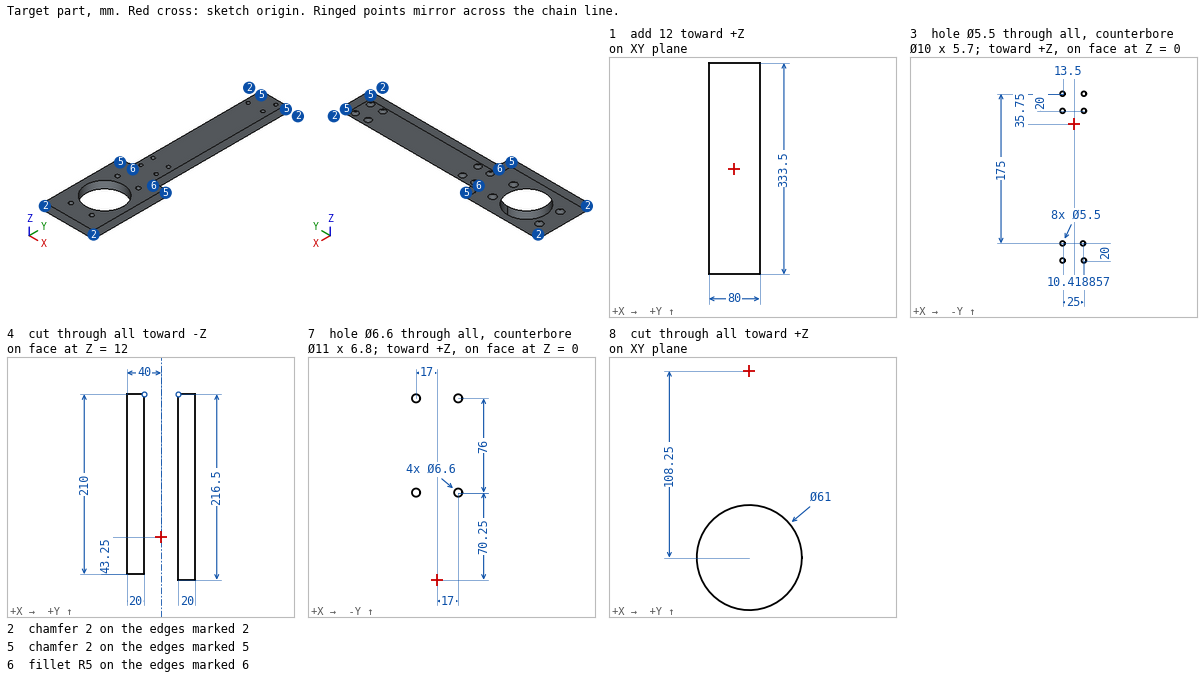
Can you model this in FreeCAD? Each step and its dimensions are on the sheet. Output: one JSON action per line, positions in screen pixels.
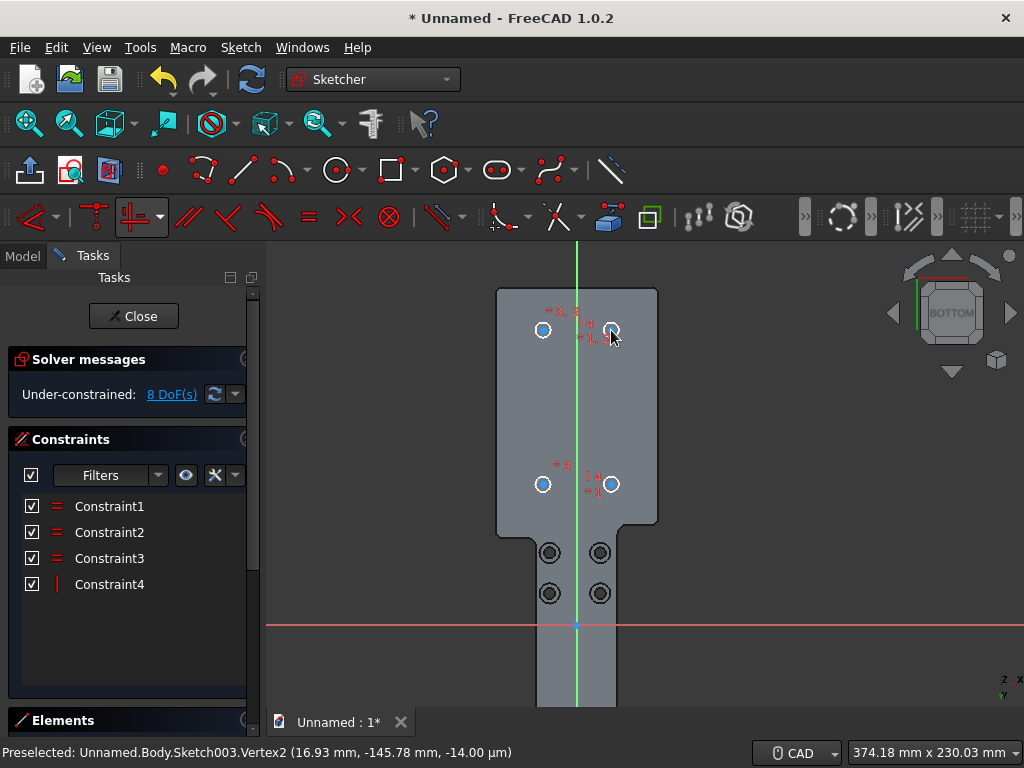
{"action": "left_click", "coordinate": [611, 330]}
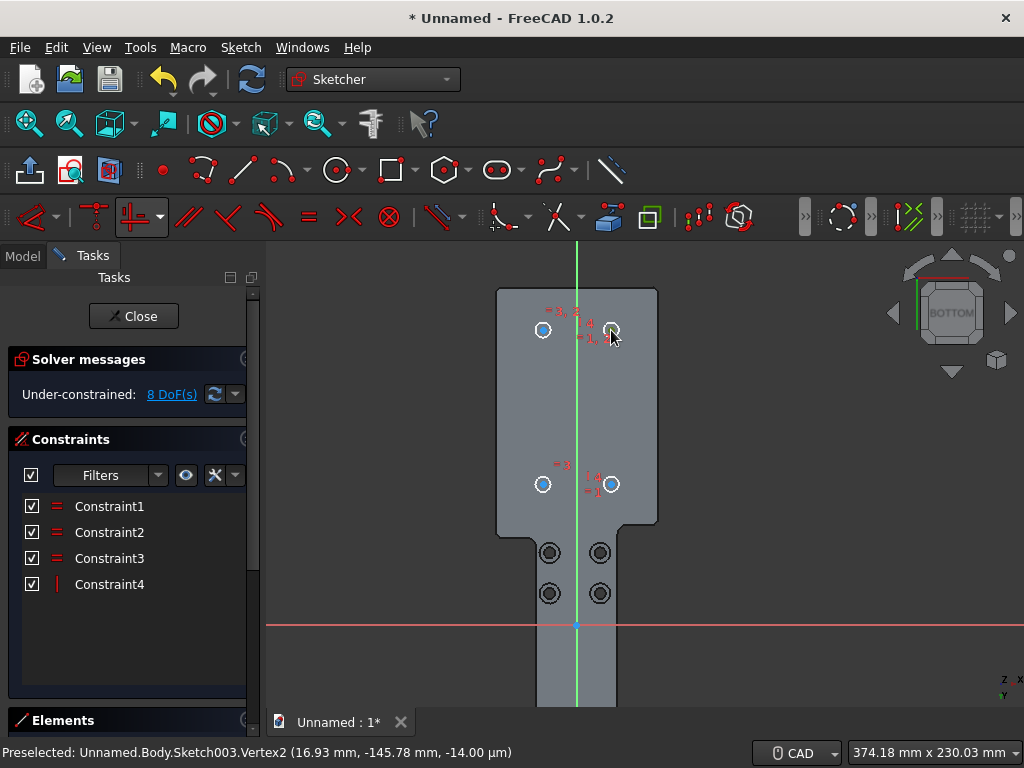
{"action": "left_click", "coordinate": [543, 330]}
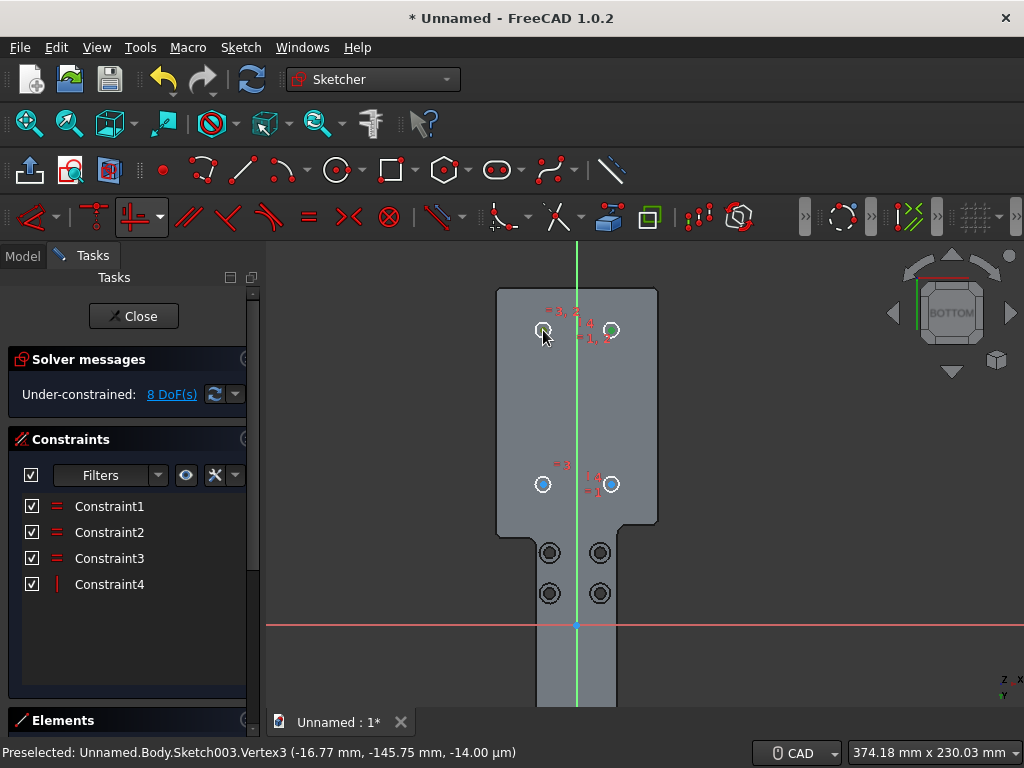
{"action": "key", "text": "h"}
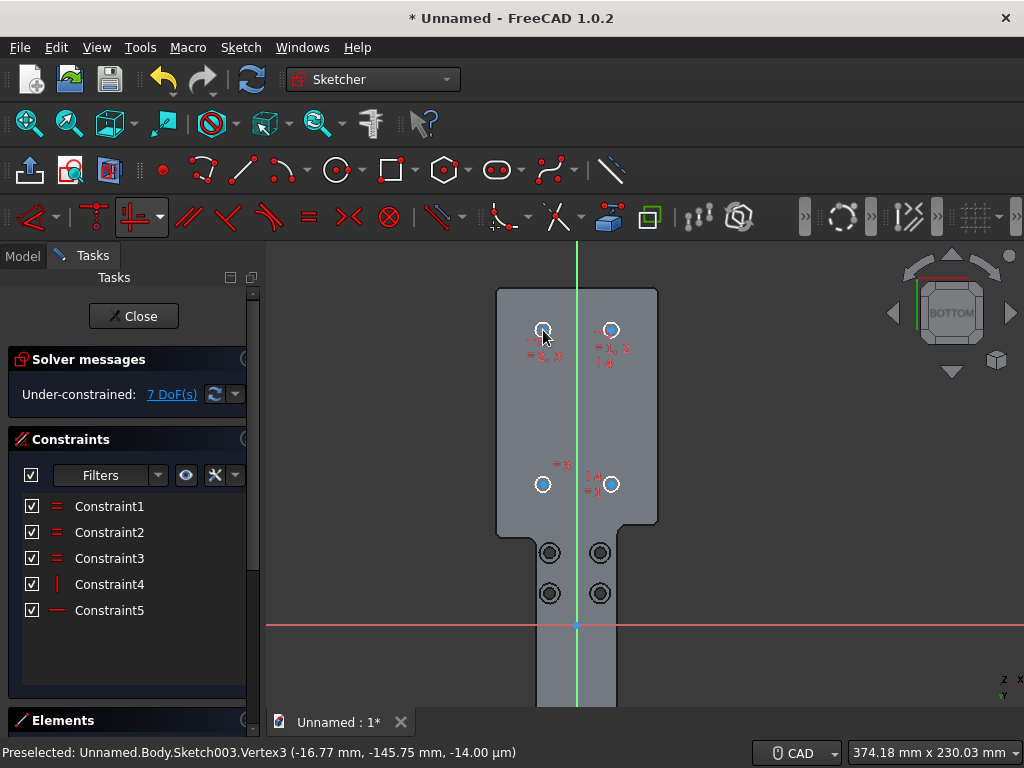
{"action": "left_click", "coordinate": [543, 330]}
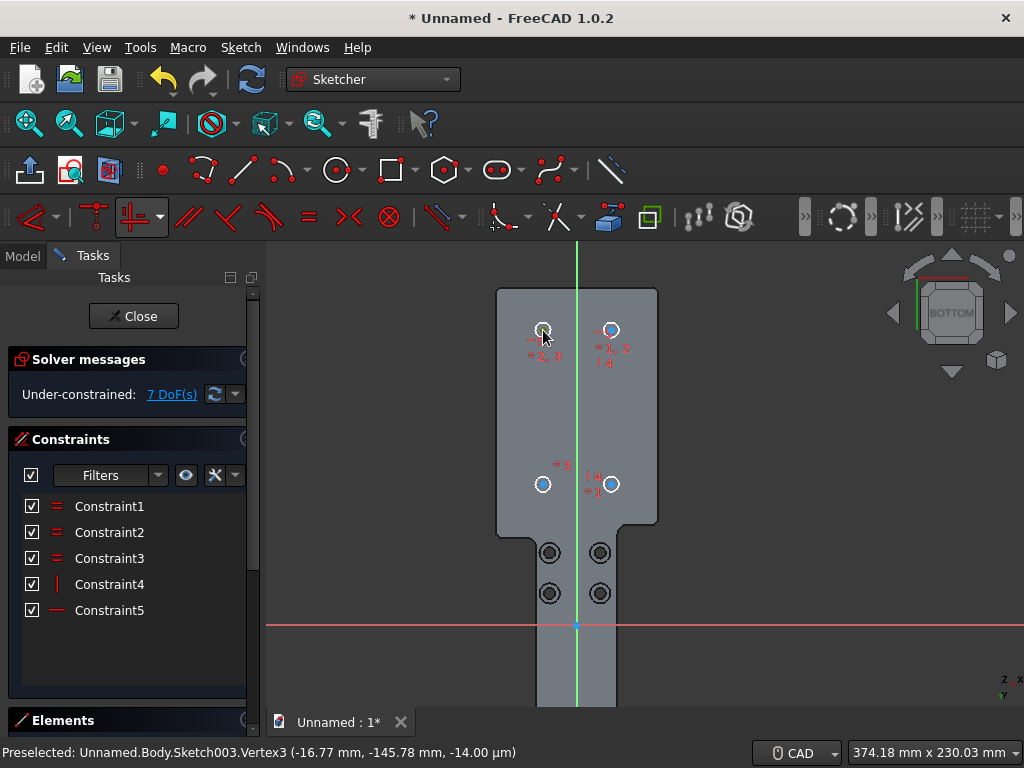
{"action": "left_click", "coordinate": [543, 484]}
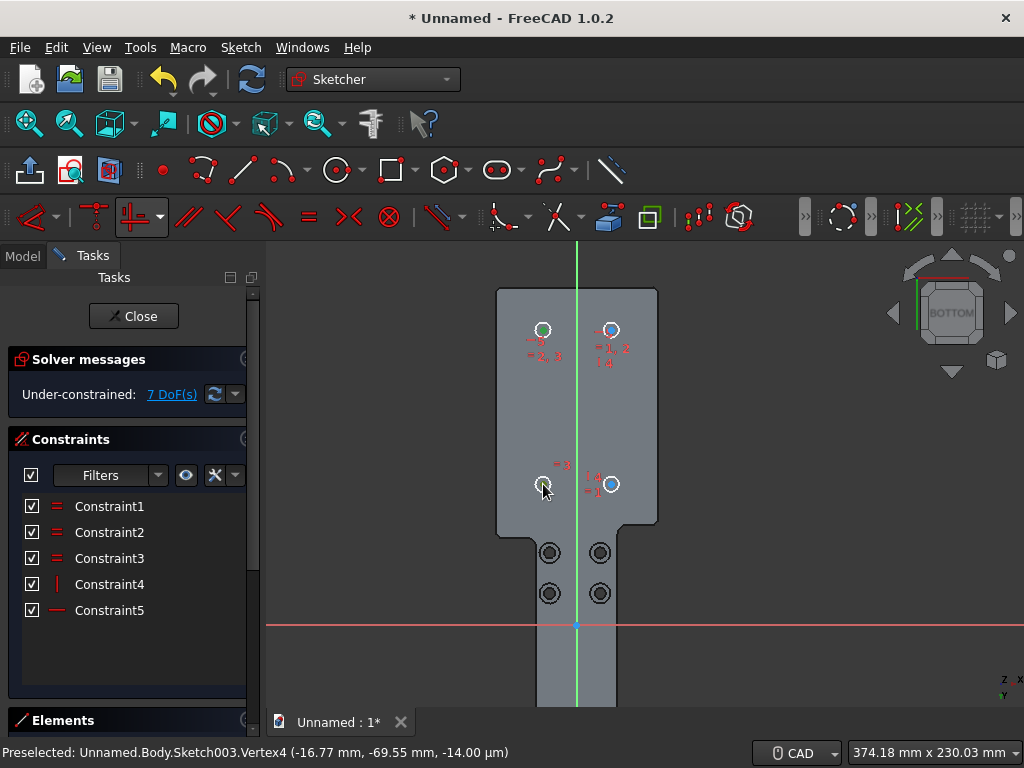
{"action": "key", "text": "v"}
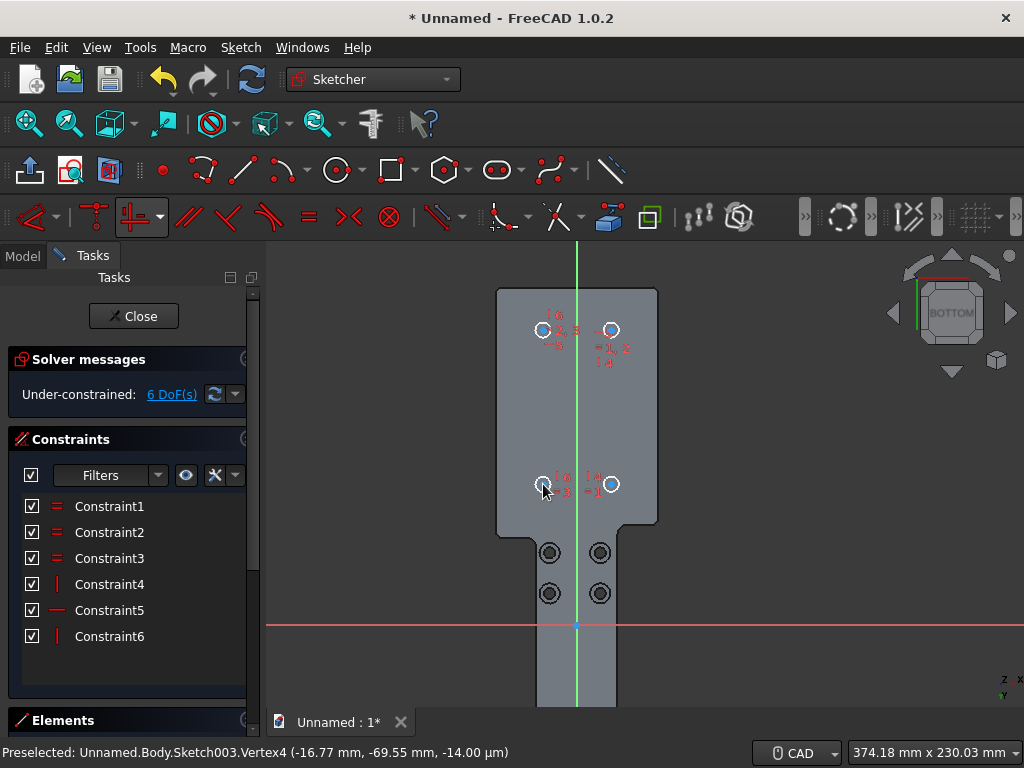
{"action": "left_click", "coordinate": [611, 484]}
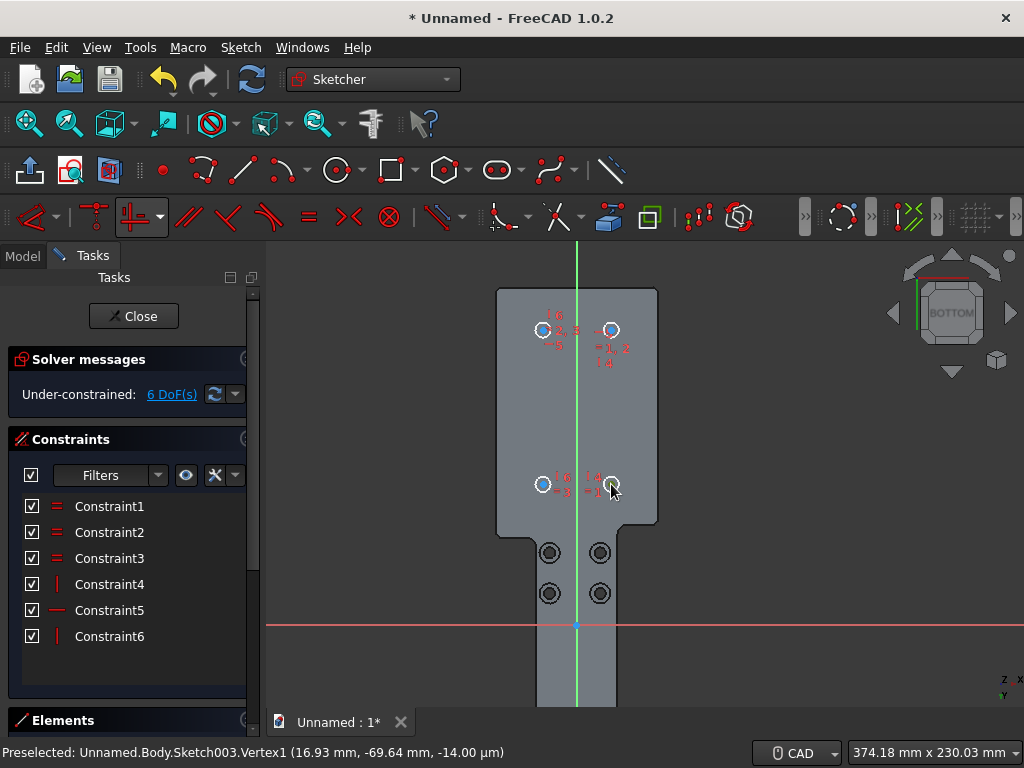
{"action": "left_click", "coordinate": [543, 484]}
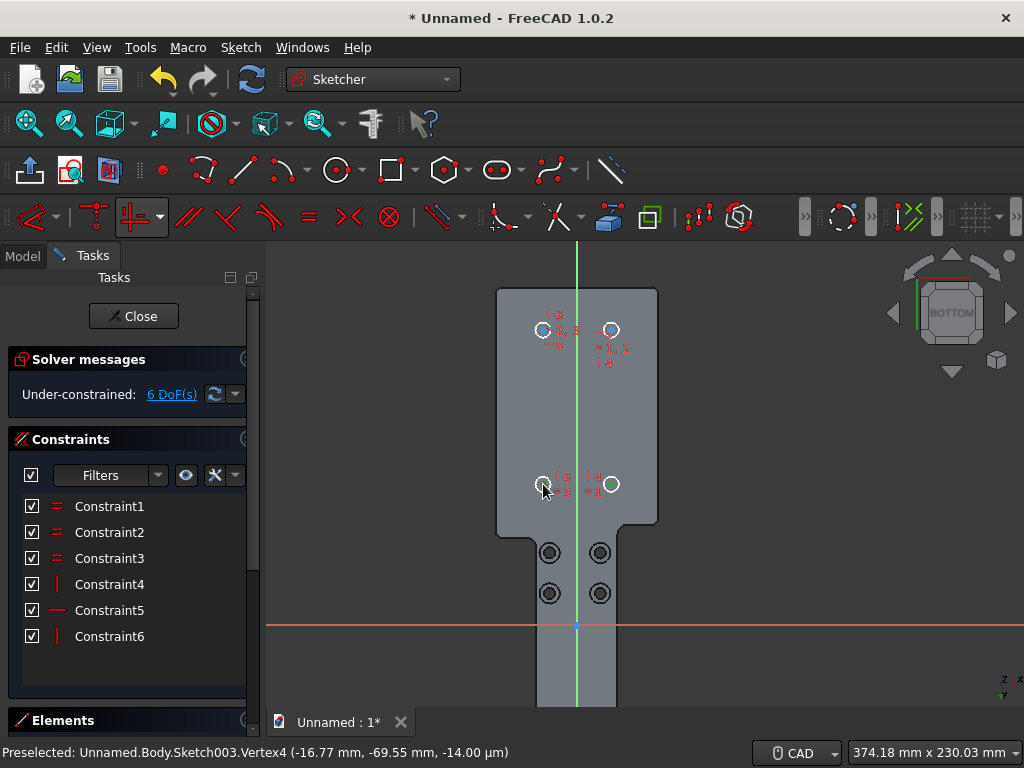
{"action": "key", "text": "h"}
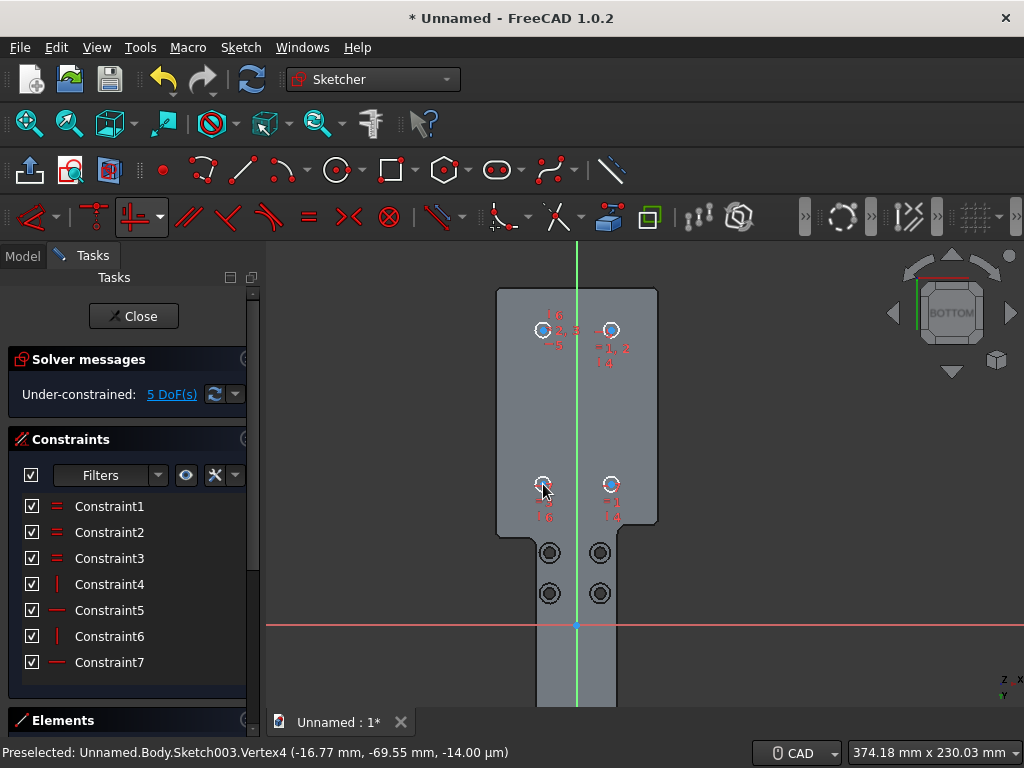
{"action": "left_click", "coordinate": [32, 218]}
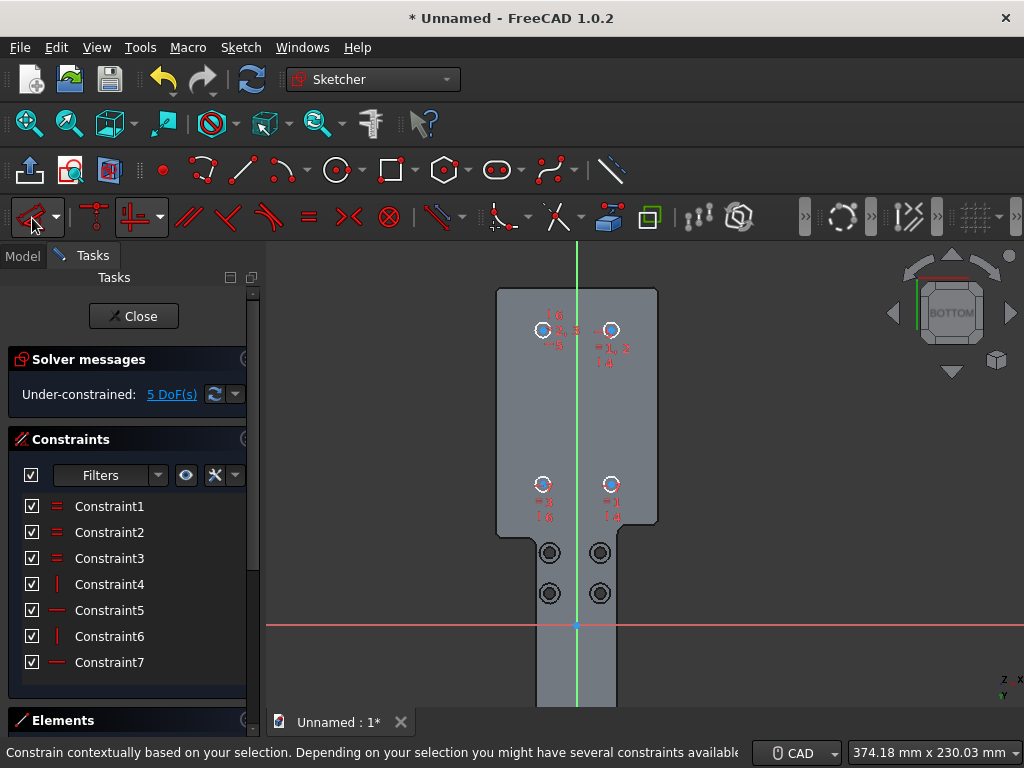
{"action": "scroll", "coordinate": [617, 490], "scroll_direction": "up", "scroll_amount": 6}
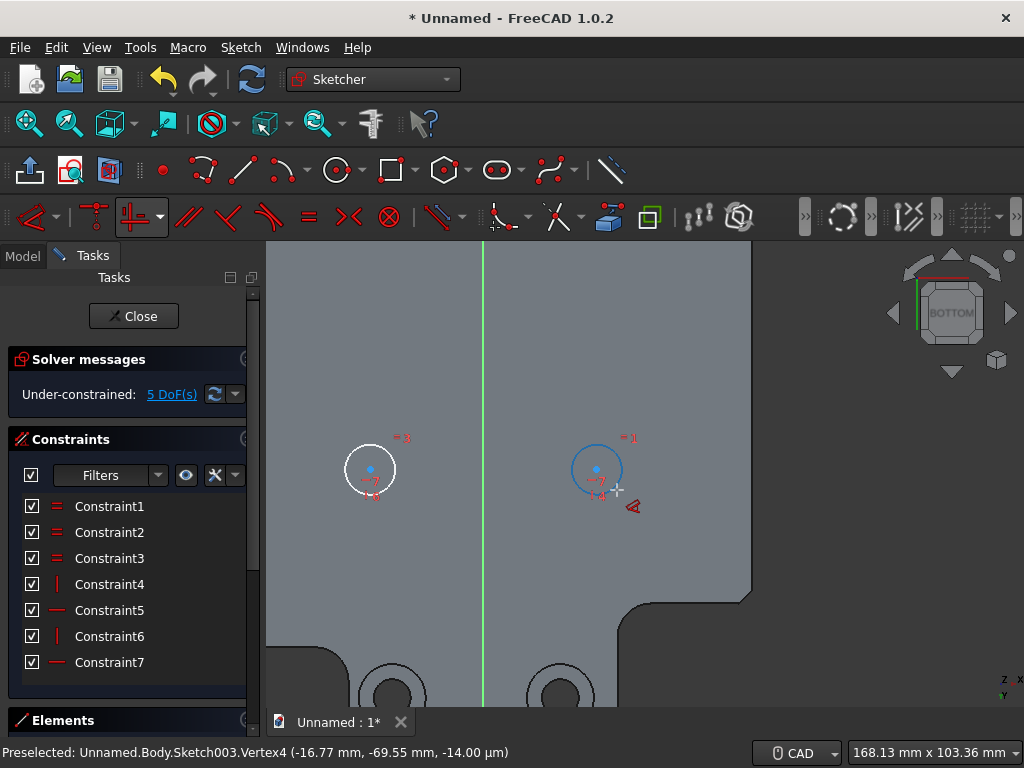
{"action": "left_click", "coordinate": [615, 487]}
{"action": "left_click", "coordinate": [638, 509]}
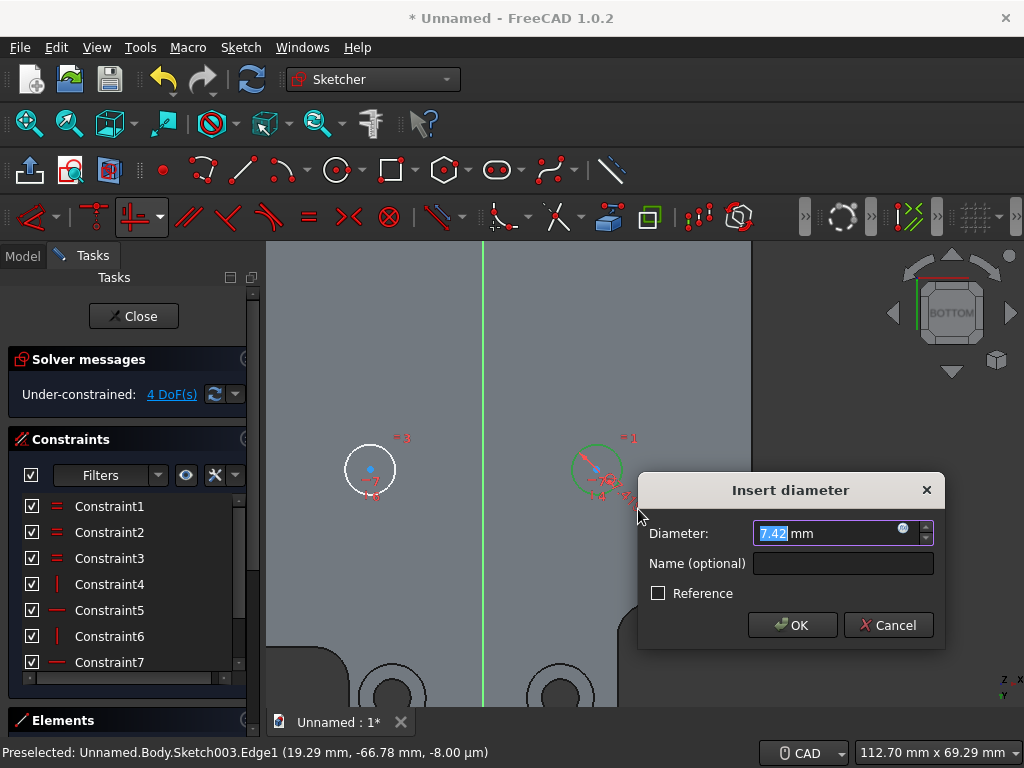
{"action": "type", "text": "6.6"}
{"action": "key", "text": "Return"}